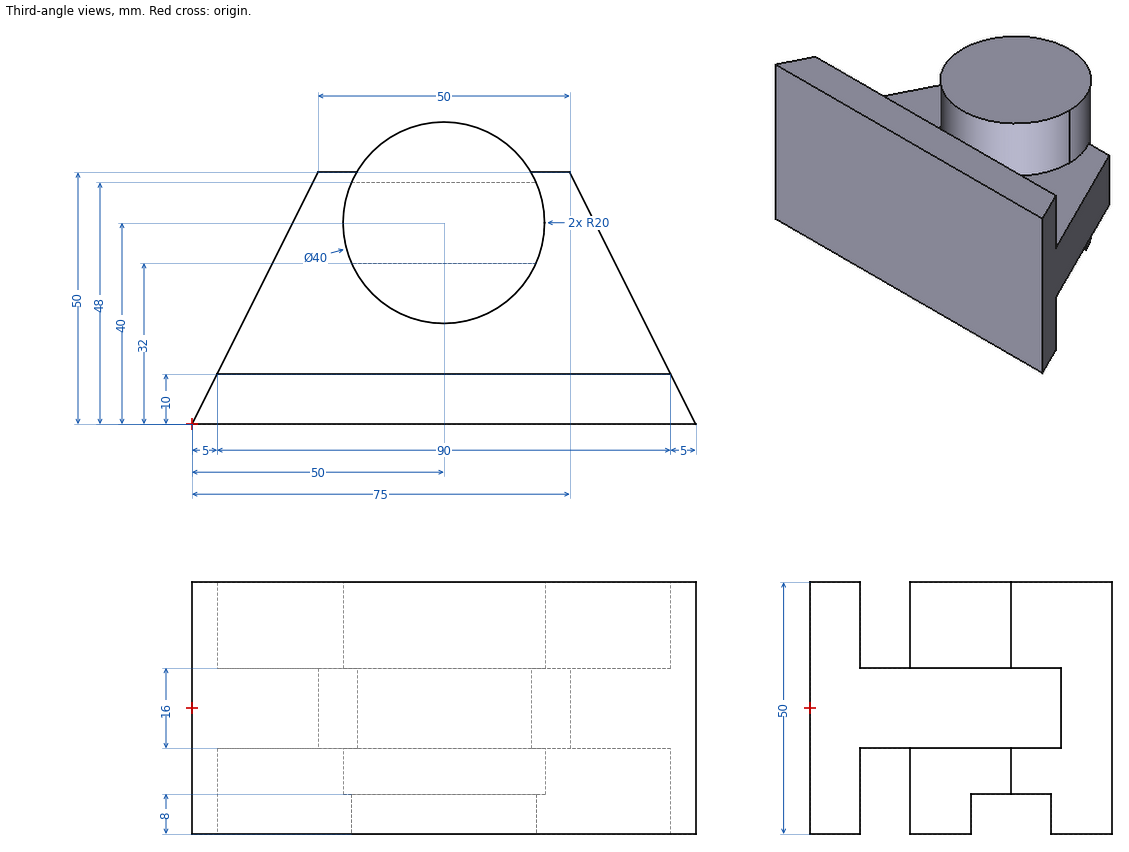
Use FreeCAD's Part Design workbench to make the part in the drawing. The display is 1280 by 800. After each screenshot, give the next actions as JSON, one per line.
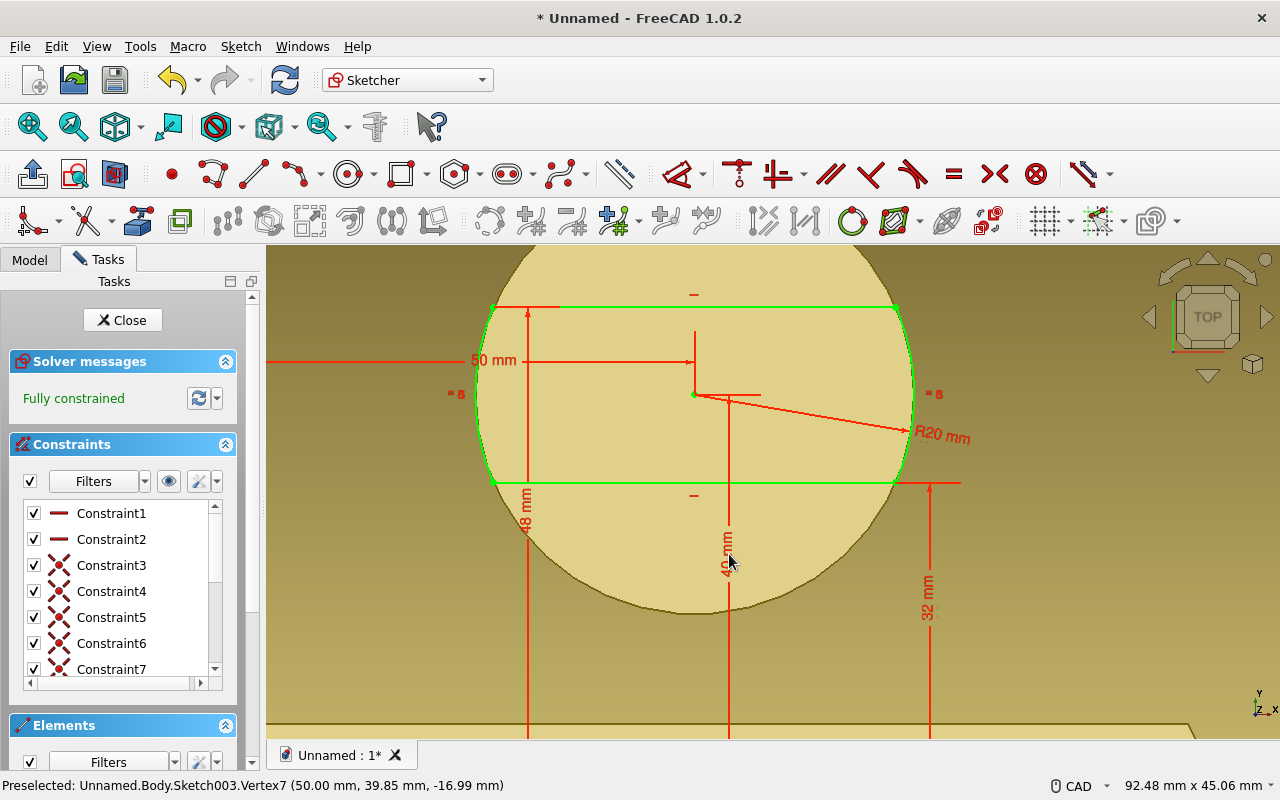
{"action": "left_click", "coordinate": [123, 320]}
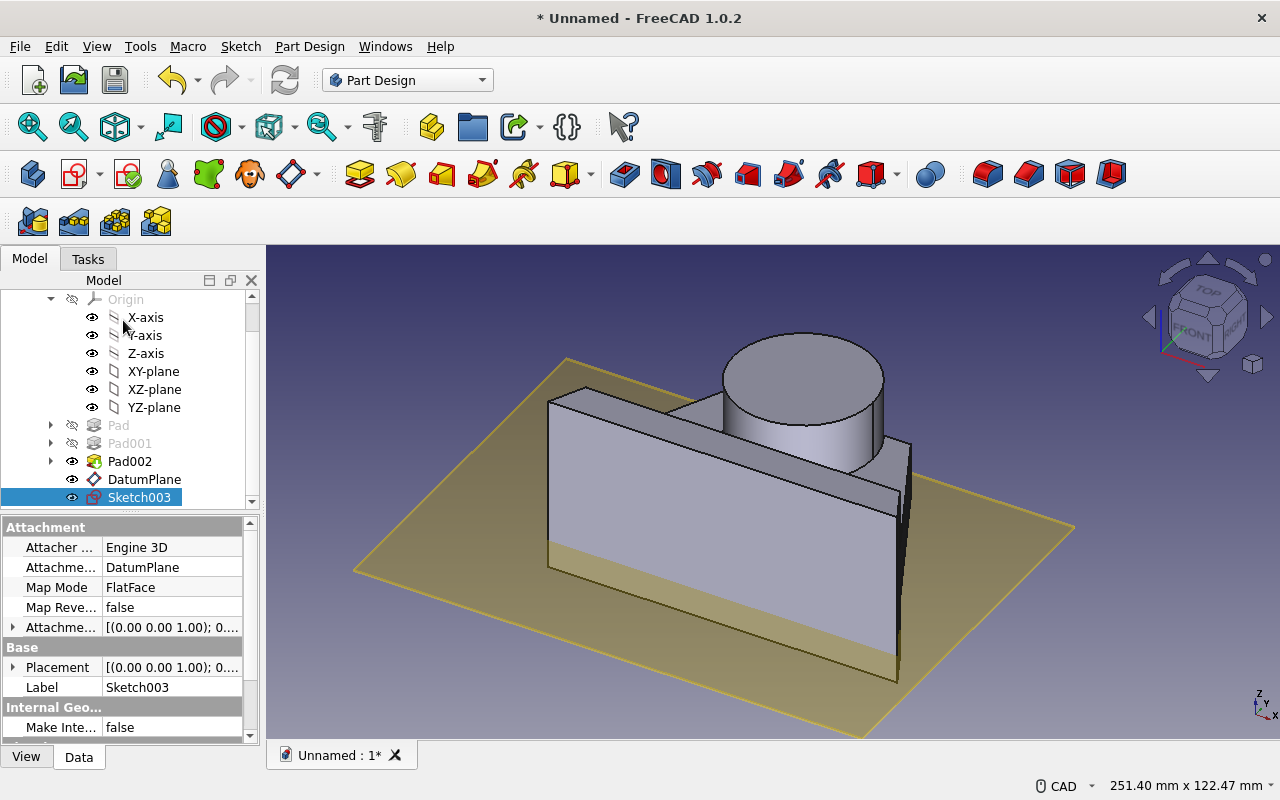
{"action": "left_click", "coordinate": [625, 174]}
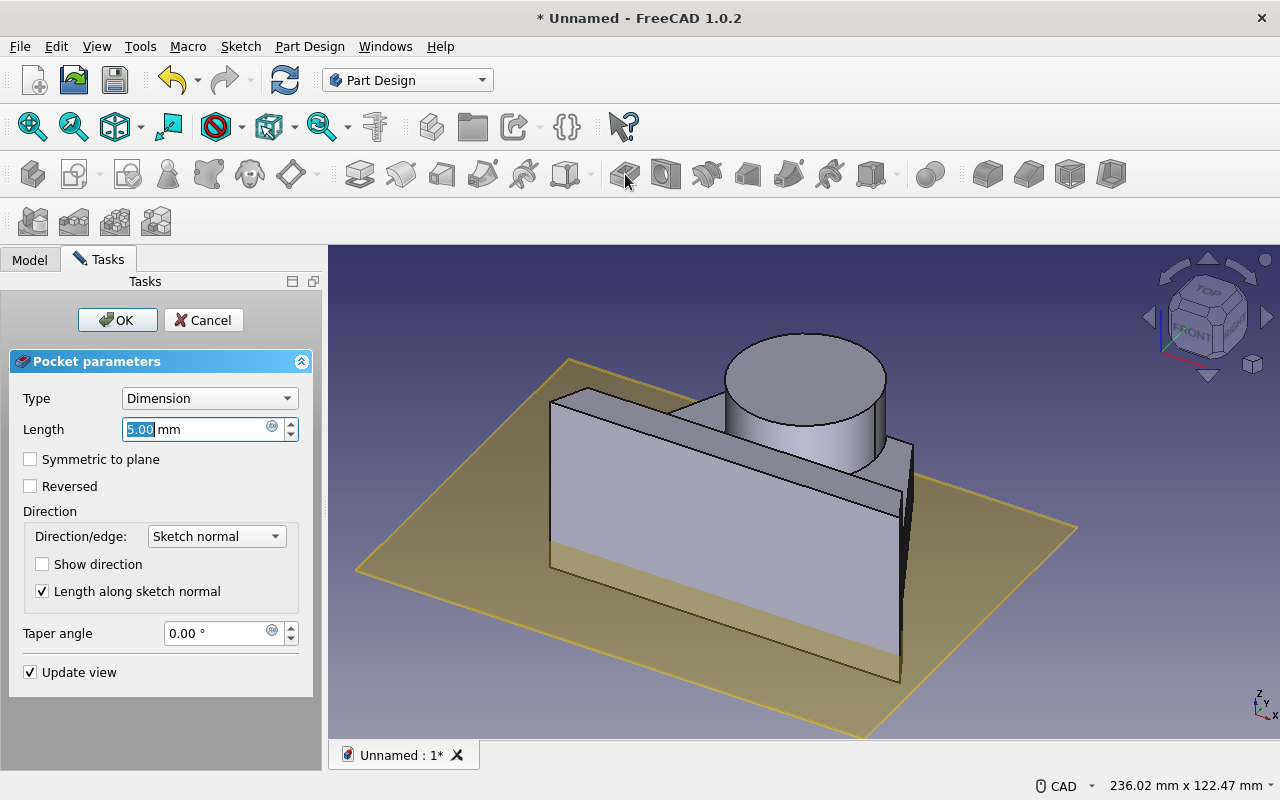
{"action": "type", "text": "8"}
{"action": "key", "text": "Tab"}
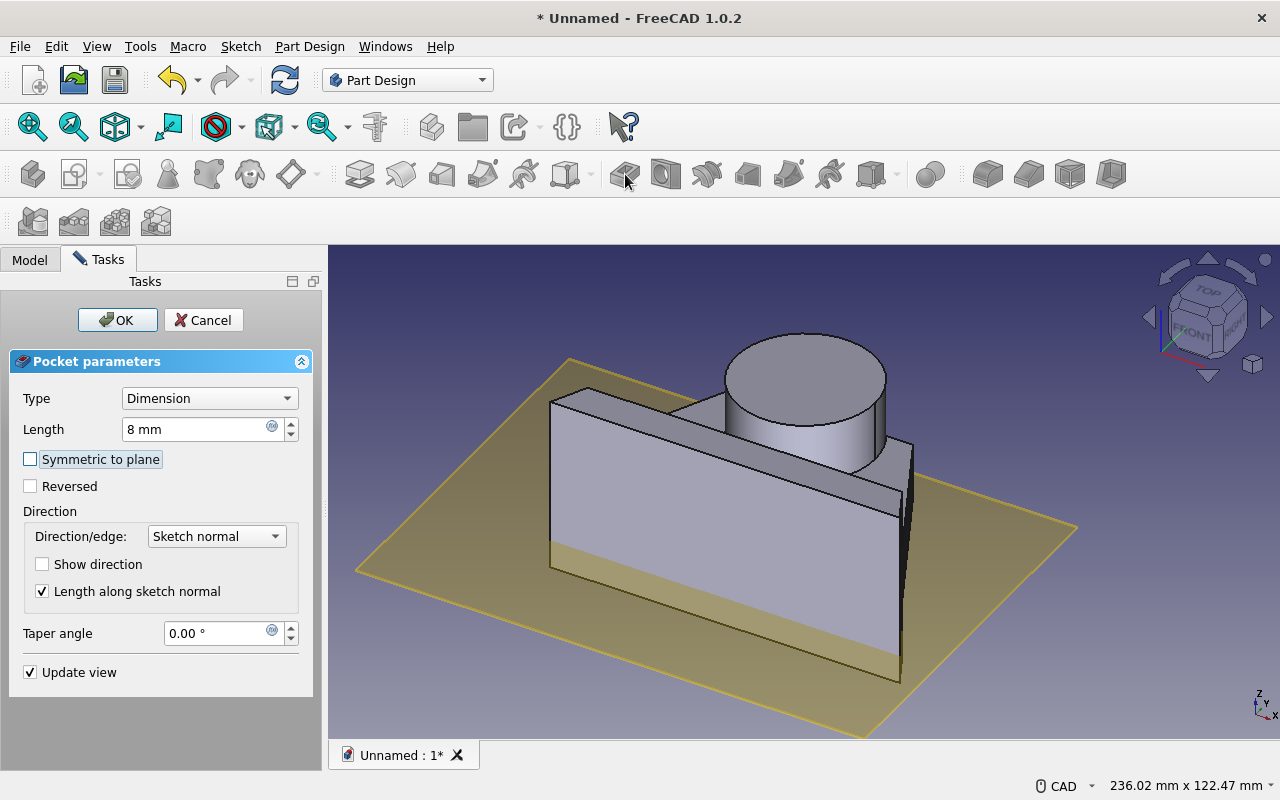
{"action": "left_click", "coordinate": [118, 320]}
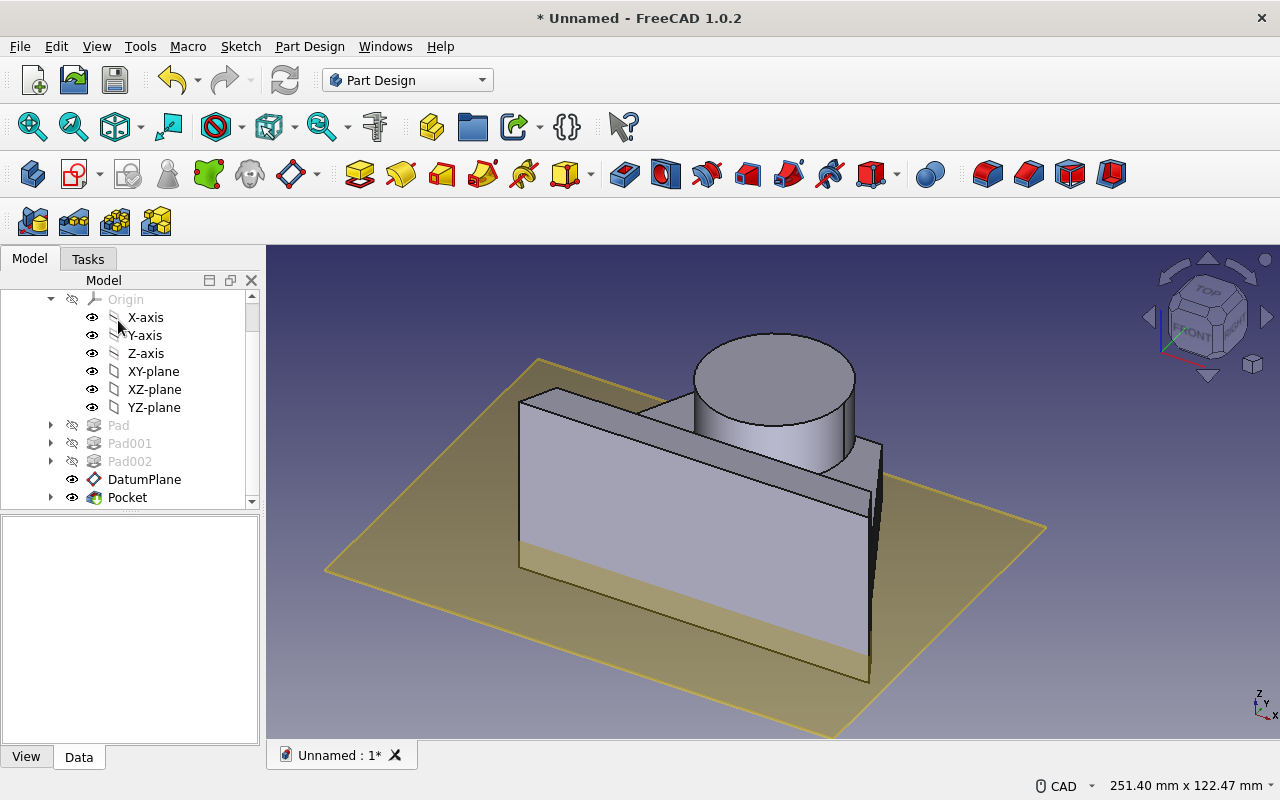
{"action": "left_click", "coordinate": [117, 479]}
{"action": "key", "text": "space"}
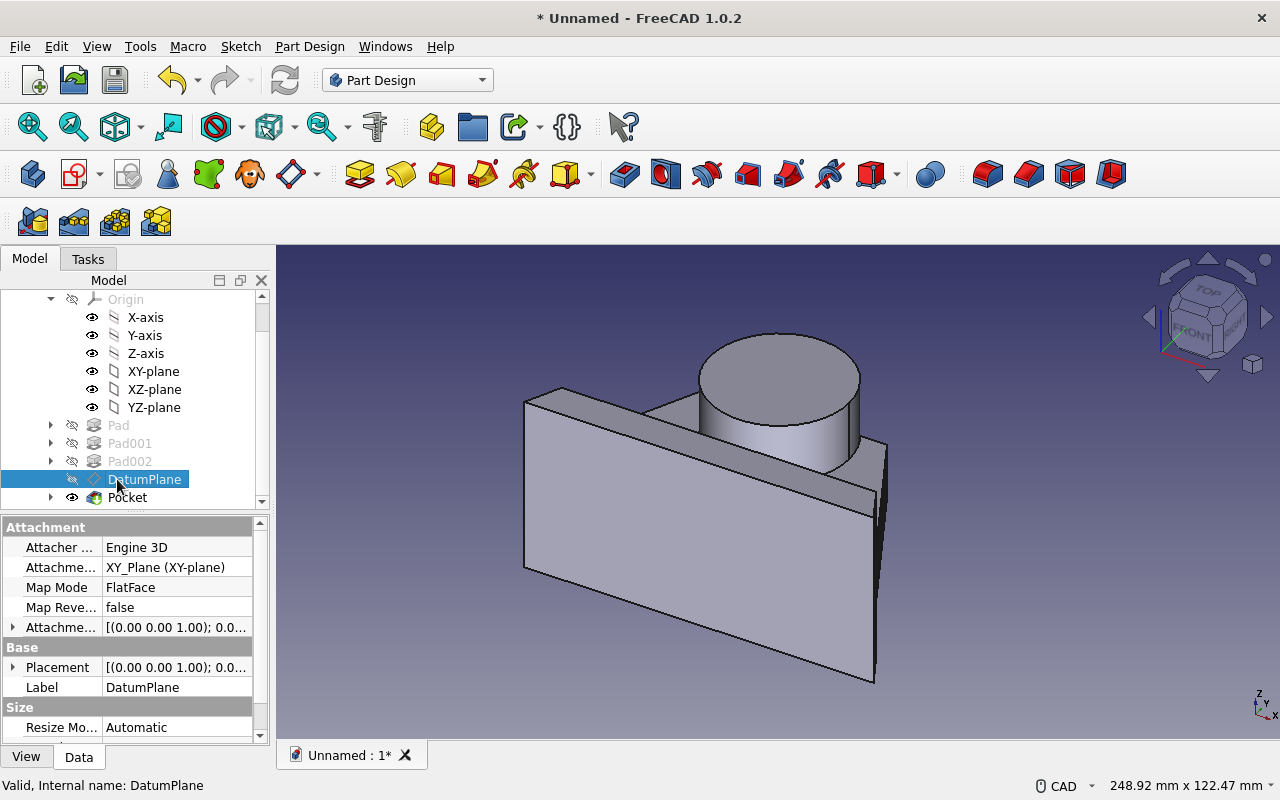
{"action": "key", "text": "0"}